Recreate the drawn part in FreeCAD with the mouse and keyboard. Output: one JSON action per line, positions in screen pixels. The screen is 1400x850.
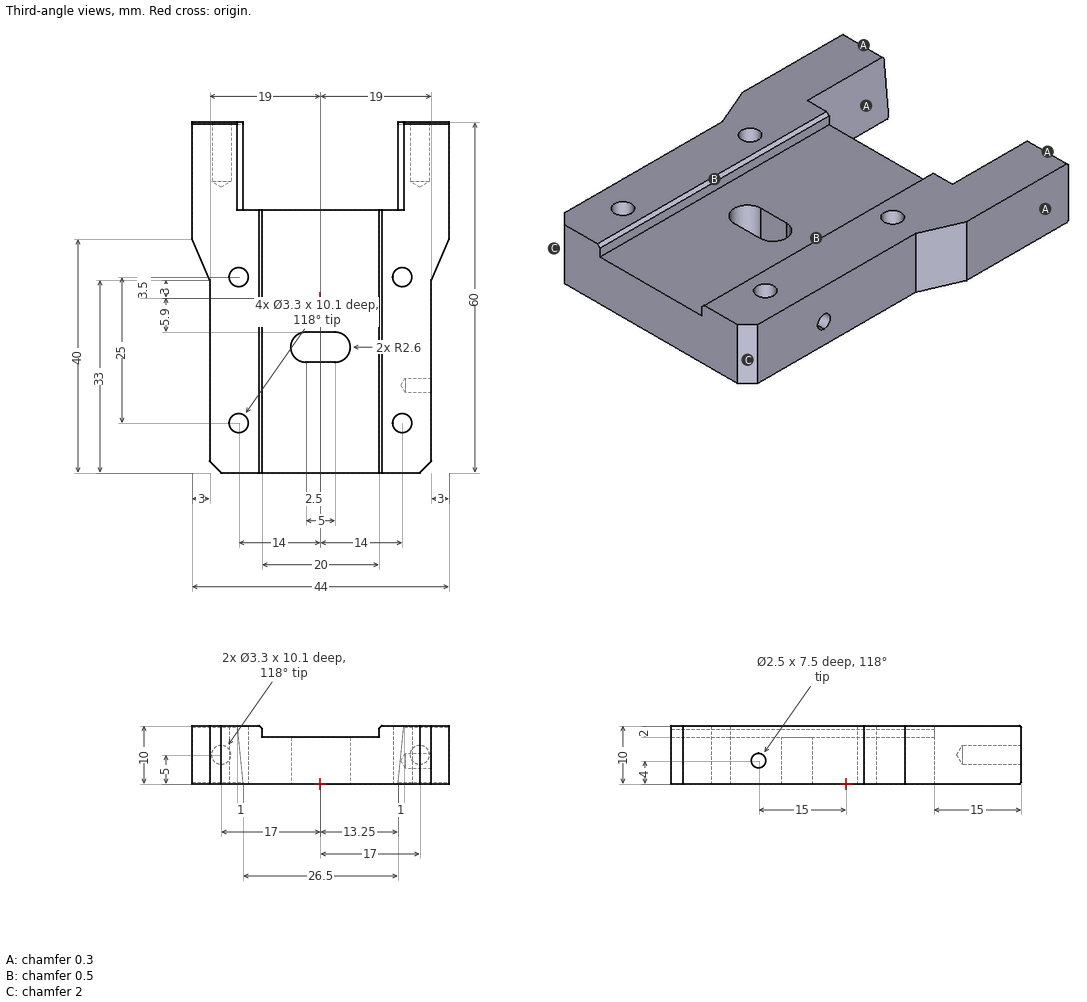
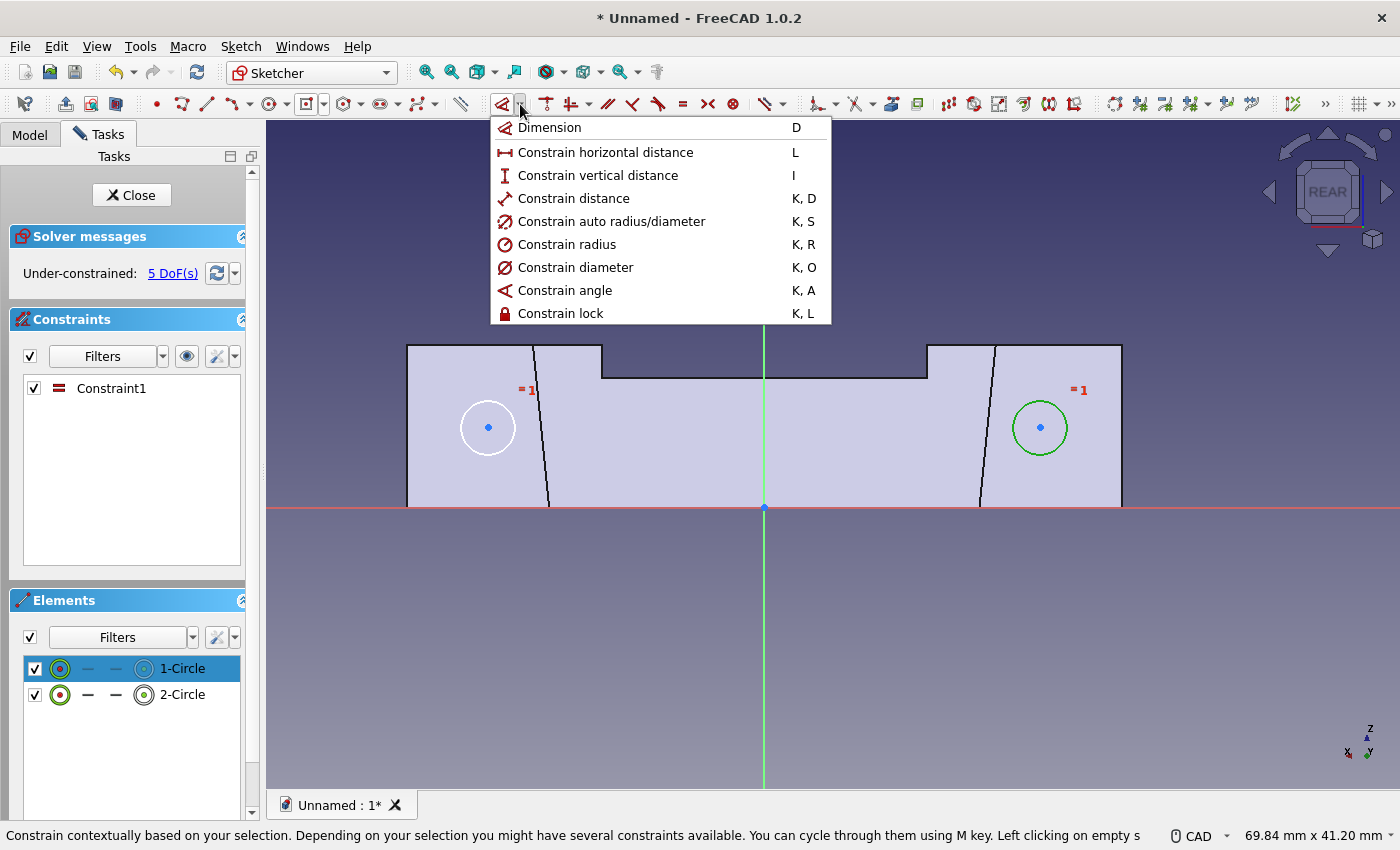
{"action": "left_click", "coordinate": [661, 268]}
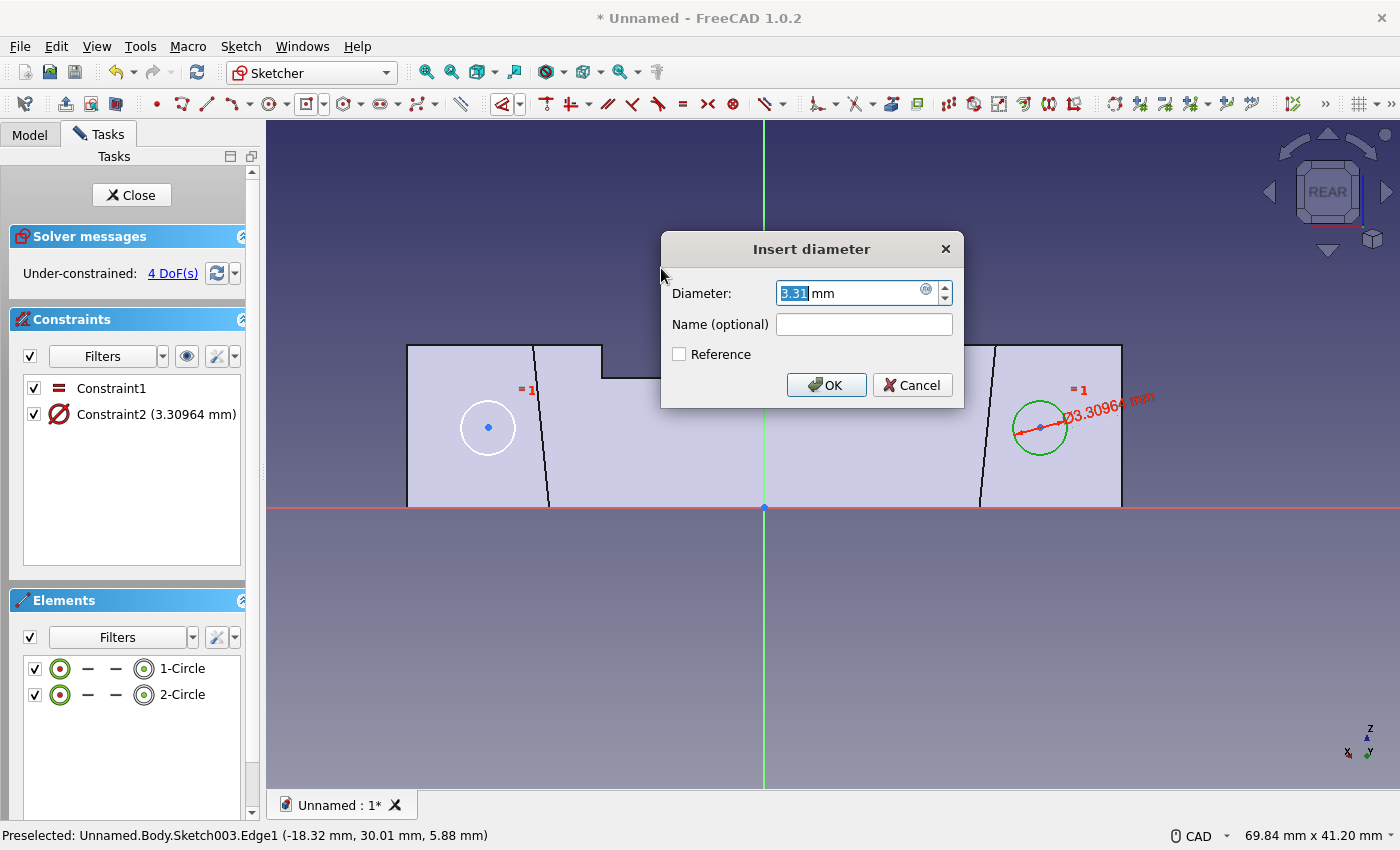
{"action": "type", "text": "3.3"}
{"action": "key", "text": "Return"}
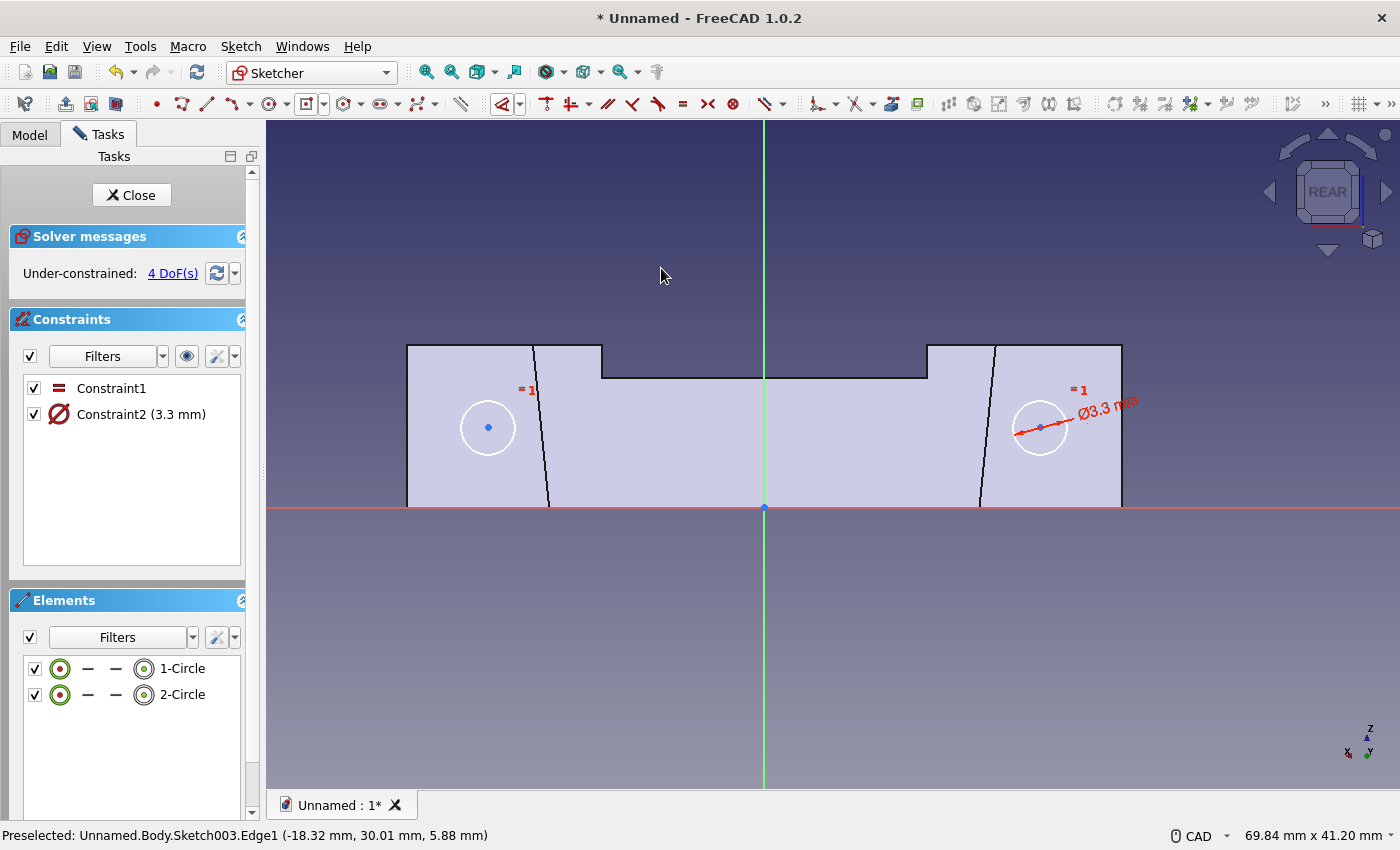
{"action": "left_click", "coordinate": [1040, 428]}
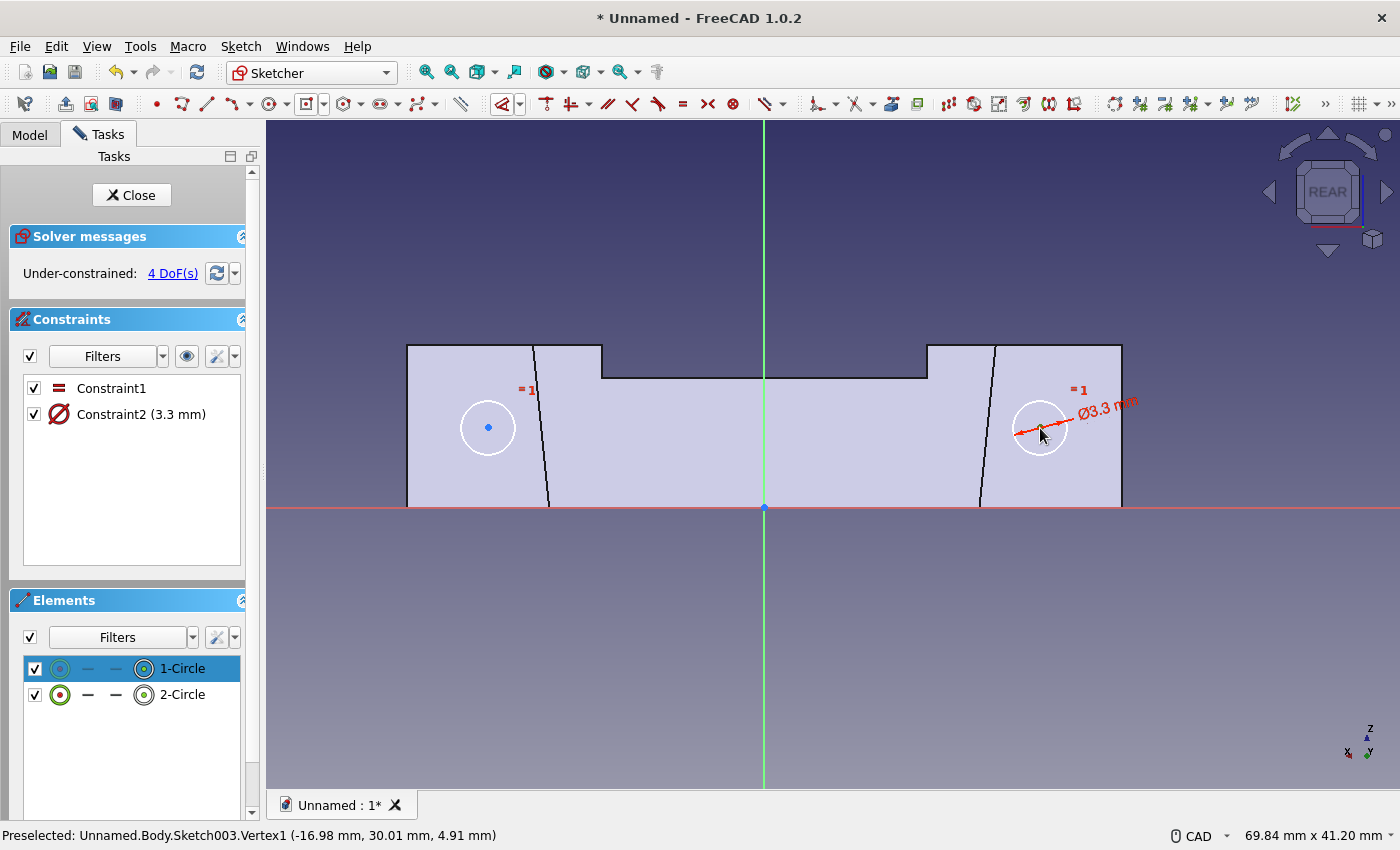
{"action": "left_click", "coordinate": [520, 104]}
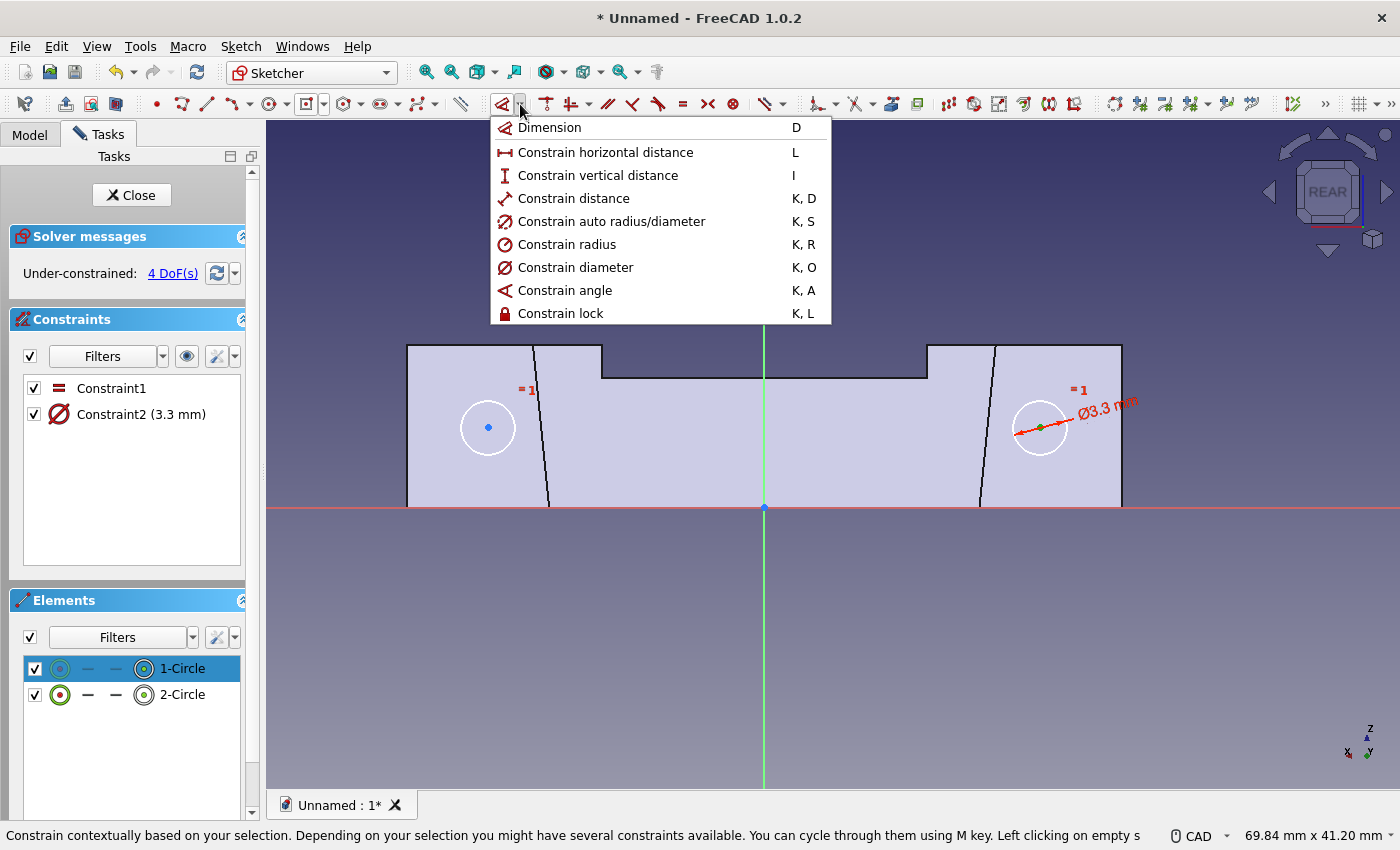
{"action": "left_click", "coordinate": [661, 176]}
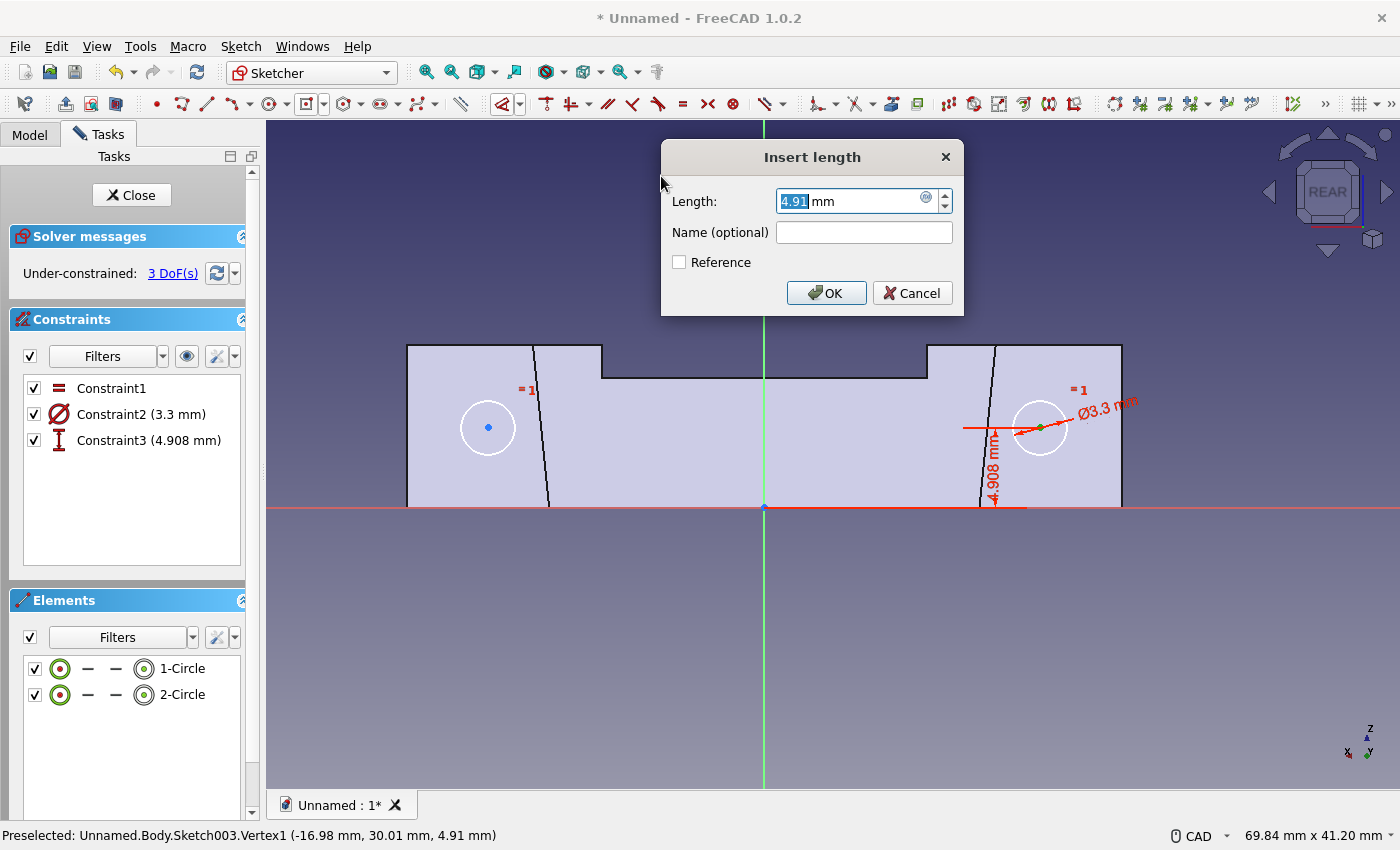
{"action": "type", "text": "5"}
{"action": "key", "text": "Return"}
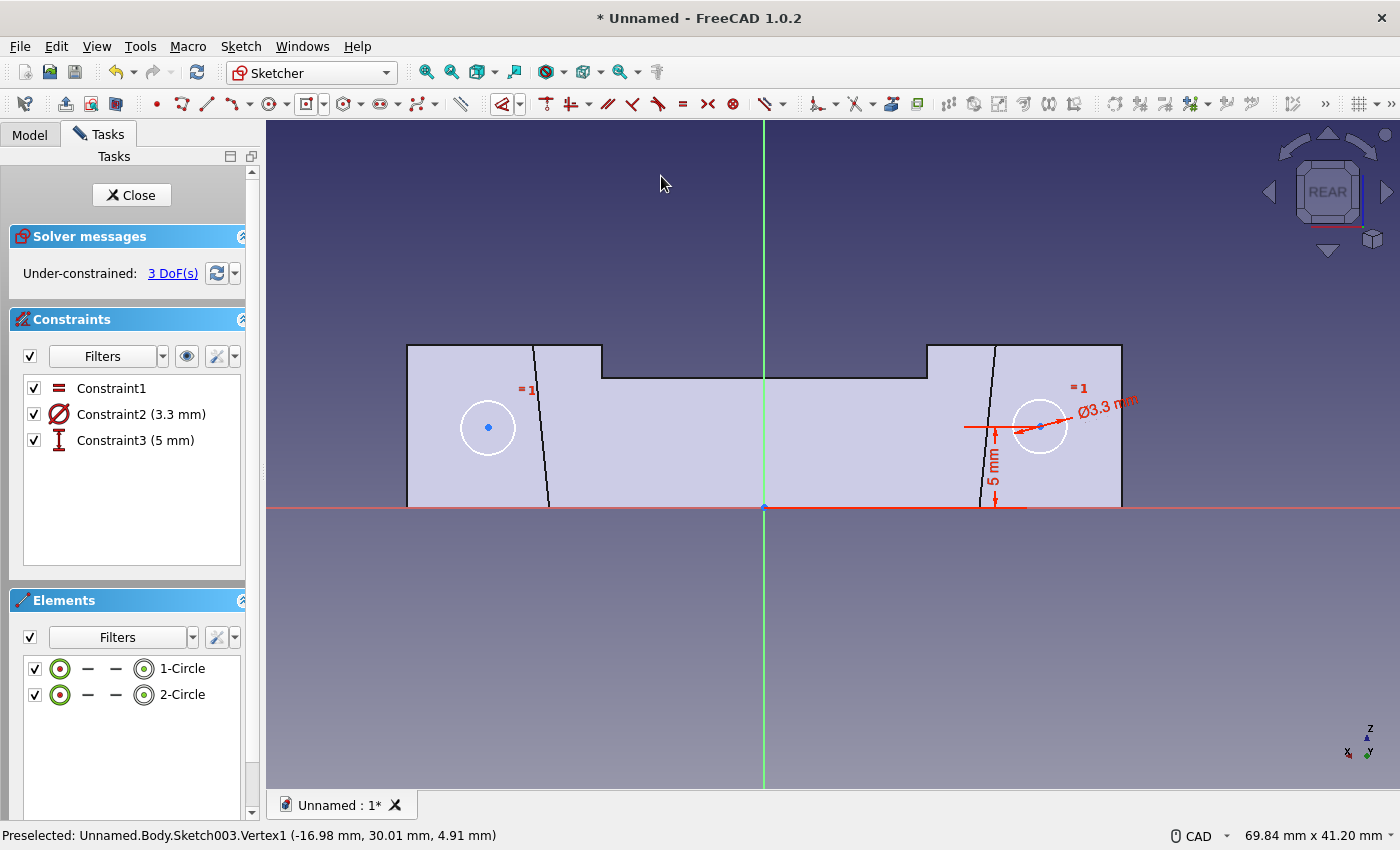
{"action": "left_click", "coordinate": [488, 428]}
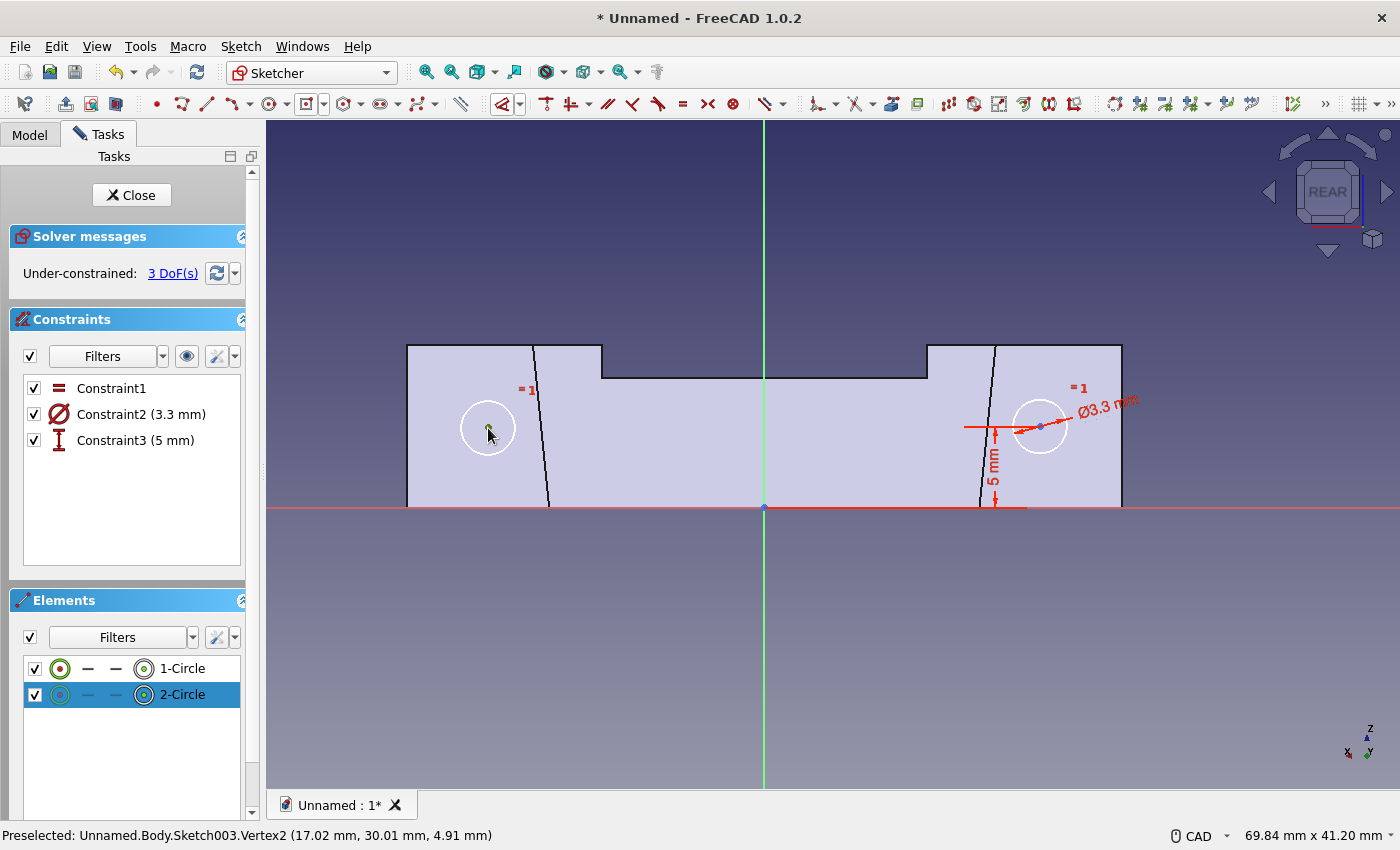
{"action": "left_click", "coordinate": [520, 104]}